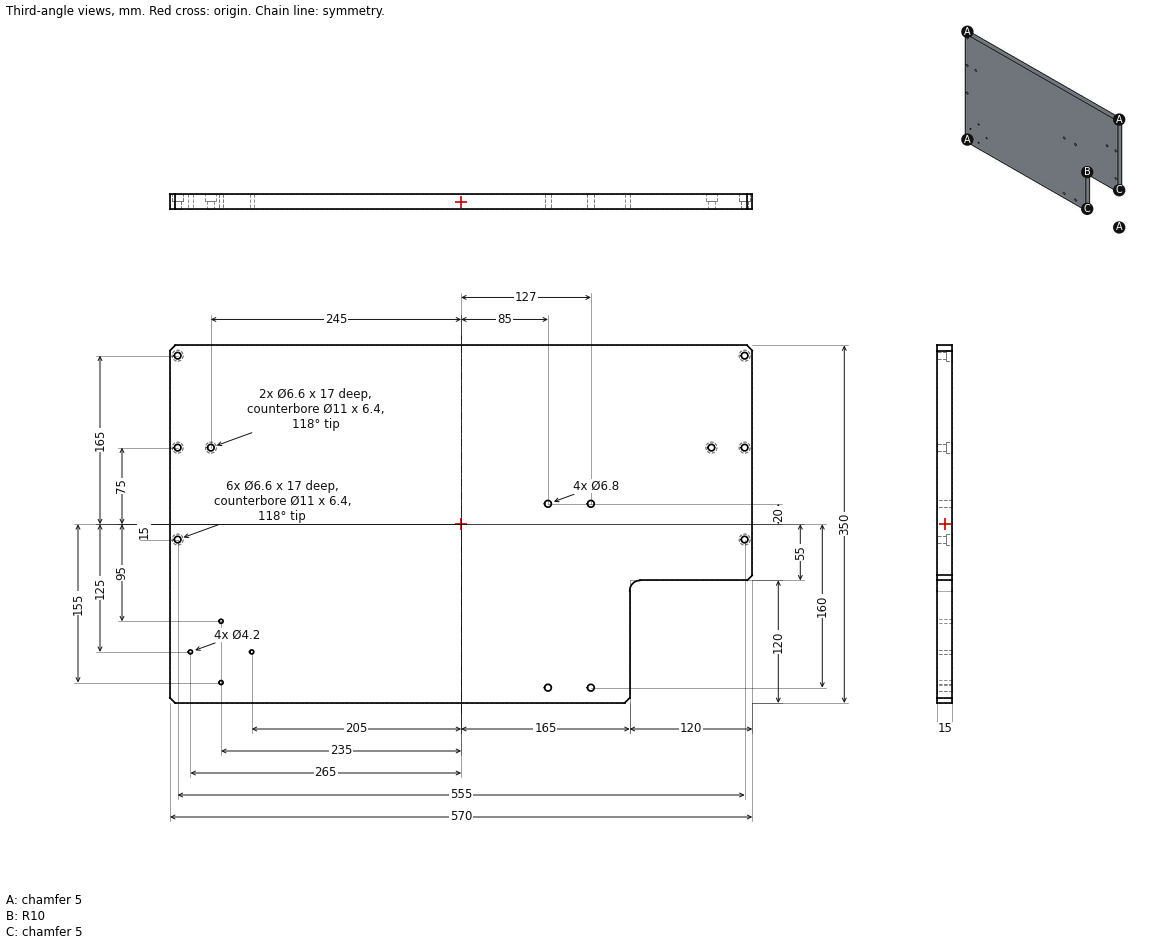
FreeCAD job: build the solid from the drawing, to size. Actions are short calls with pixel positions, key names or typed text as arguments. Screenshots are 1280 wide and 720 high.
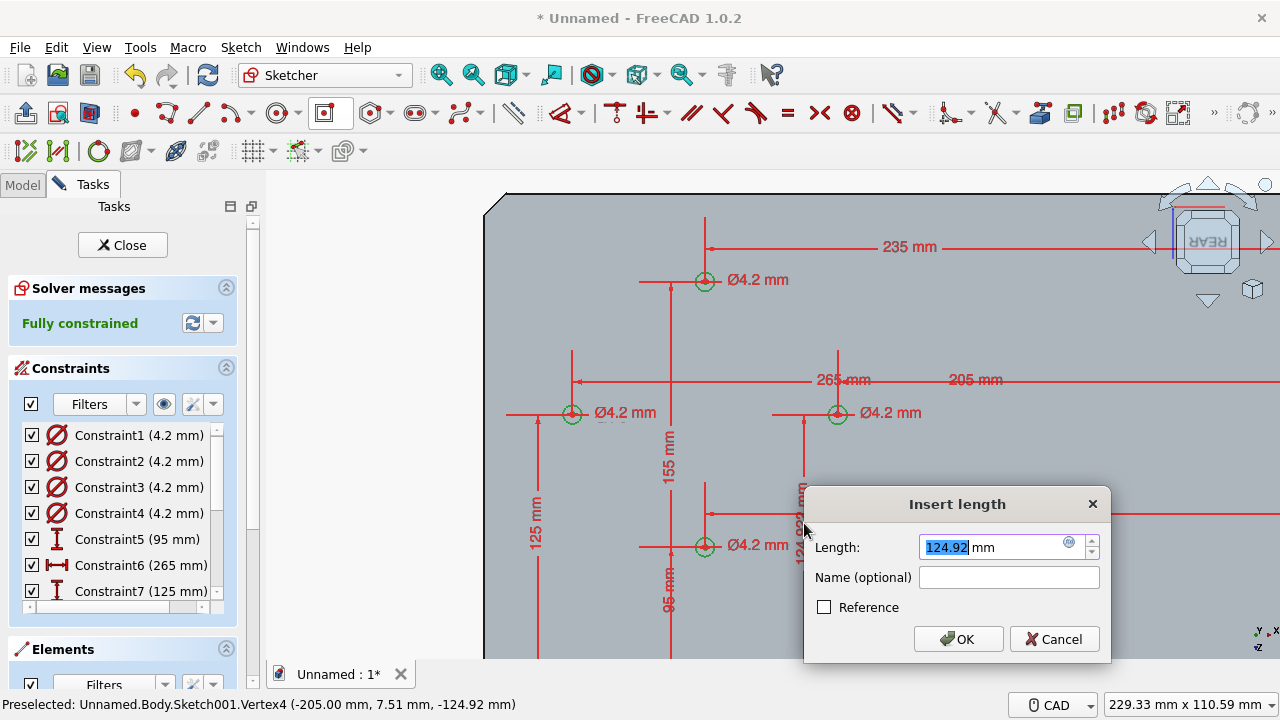
text(125)
key(Return)
key(Escape)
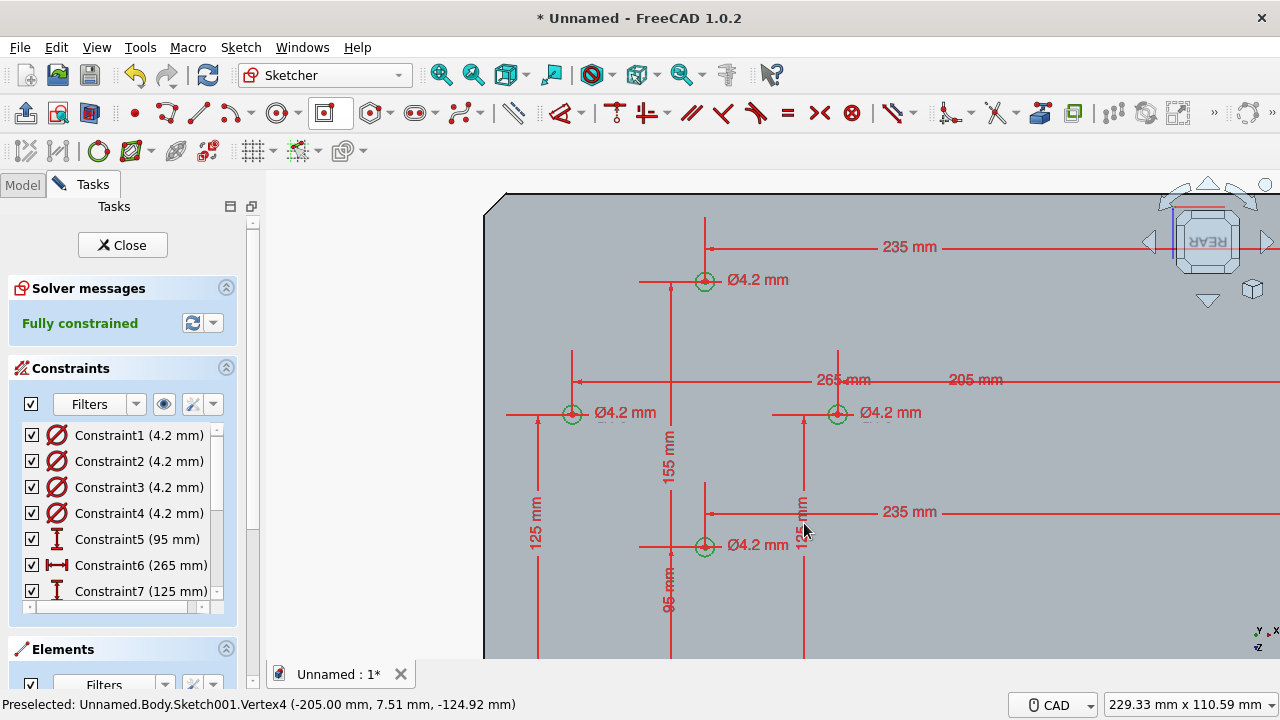
click(123, 245)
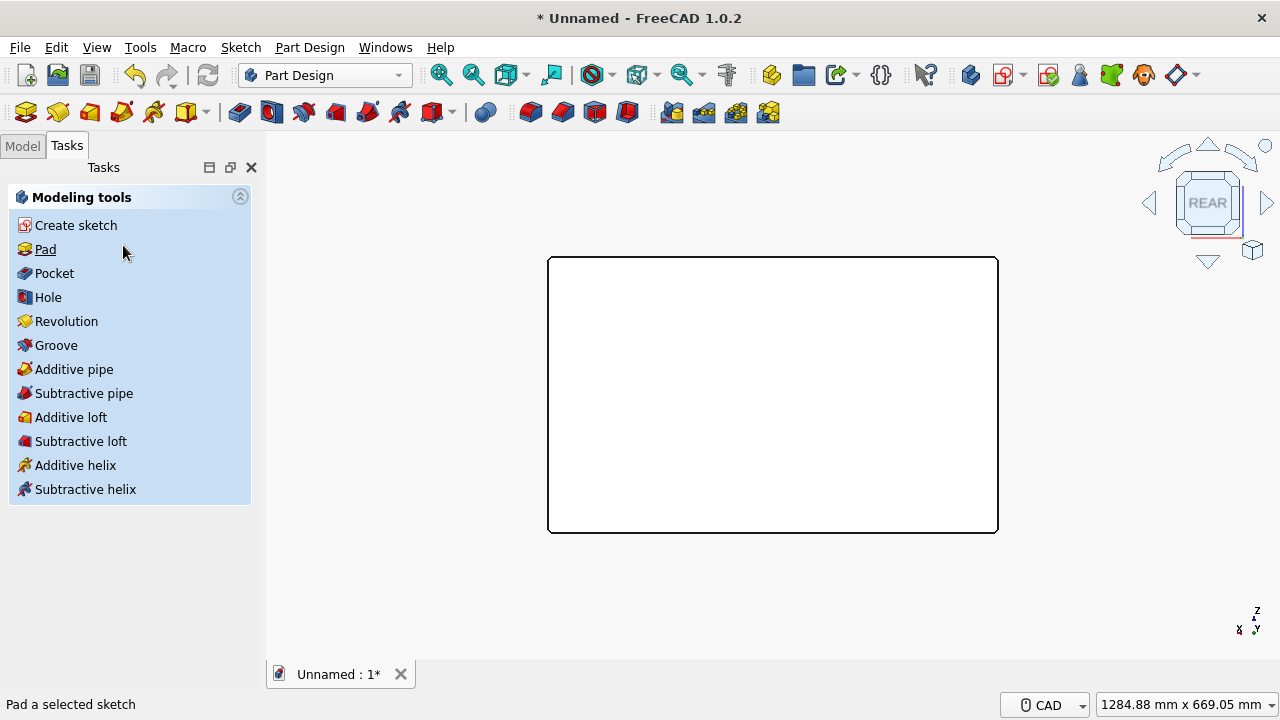
click(240, 112)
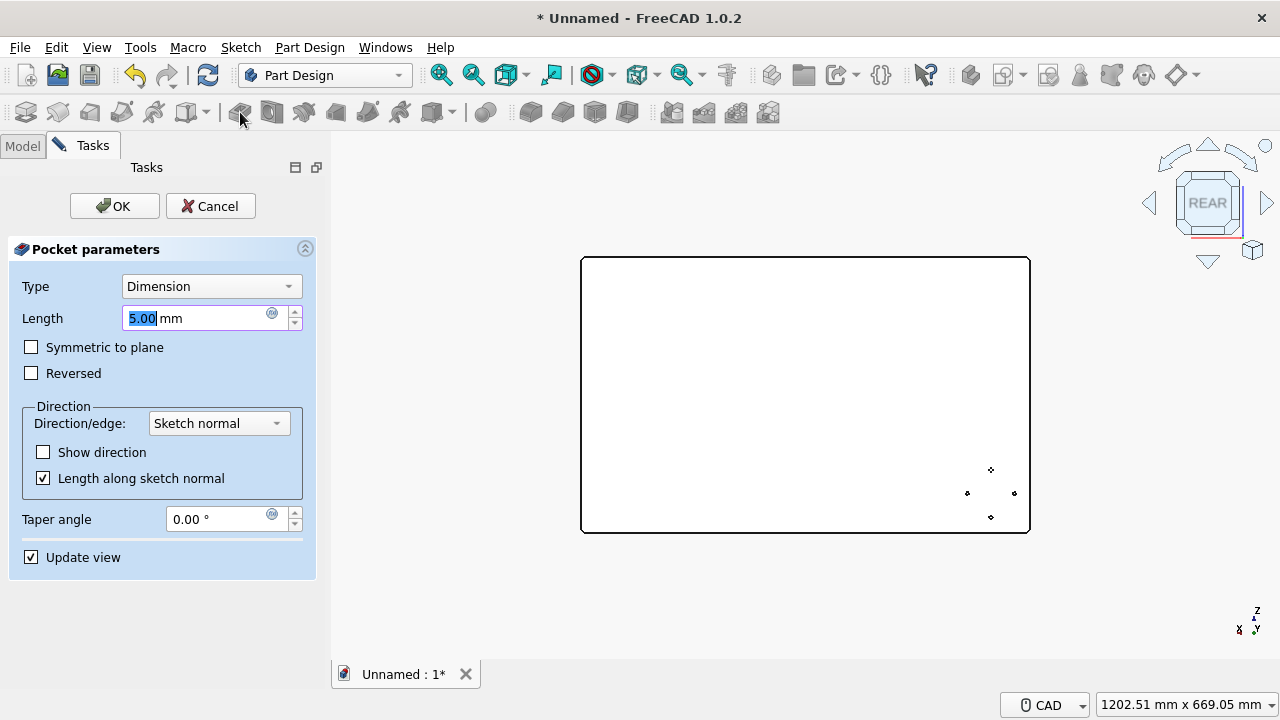
click(212, 286)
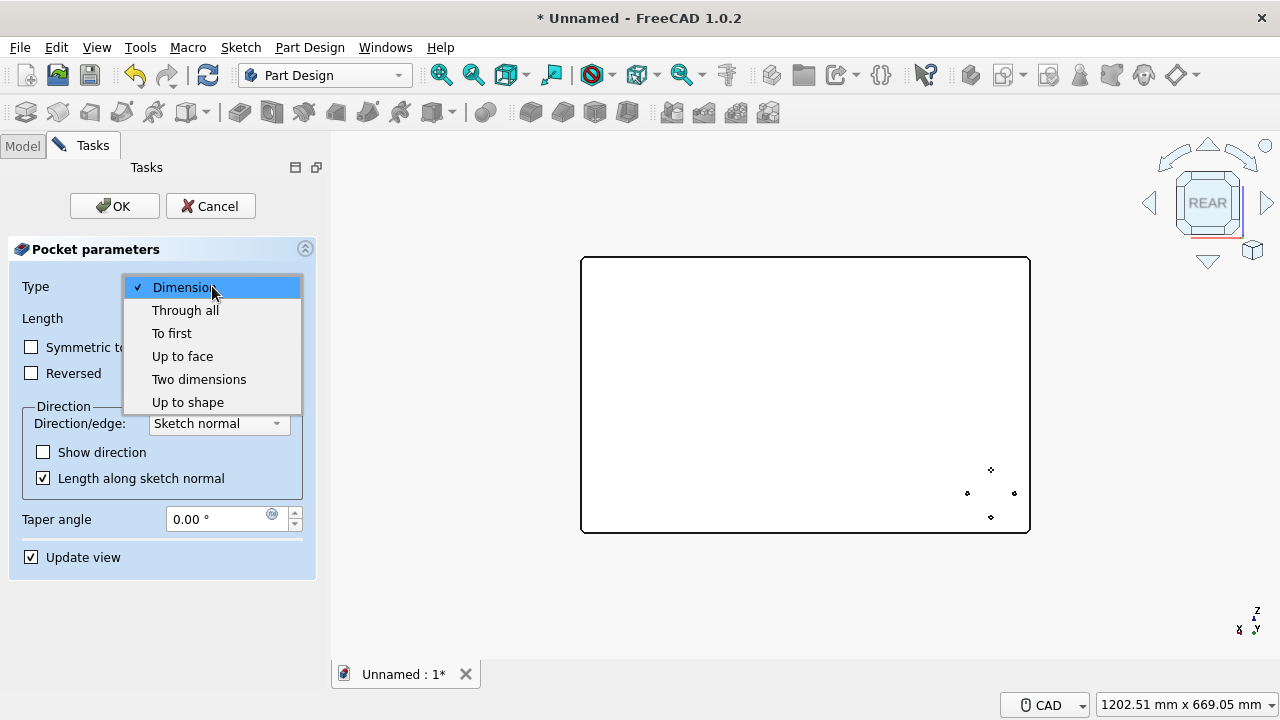
click(212, 310)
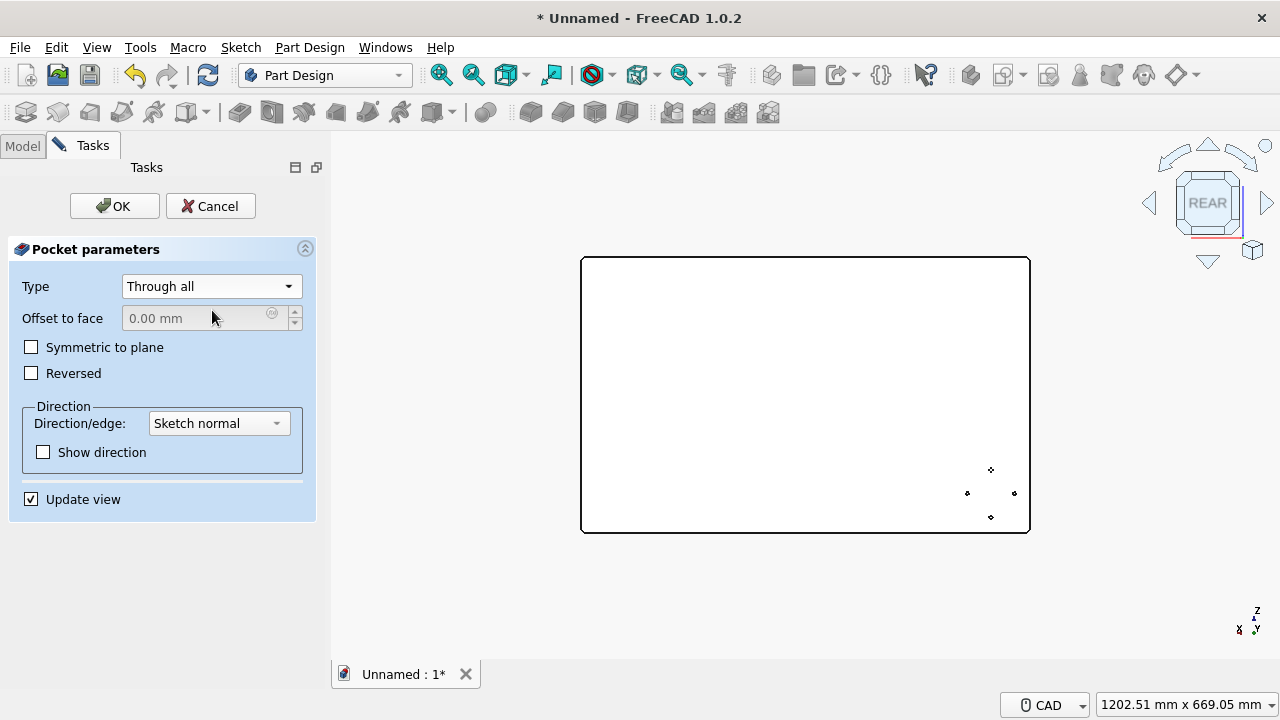
click(115, 206)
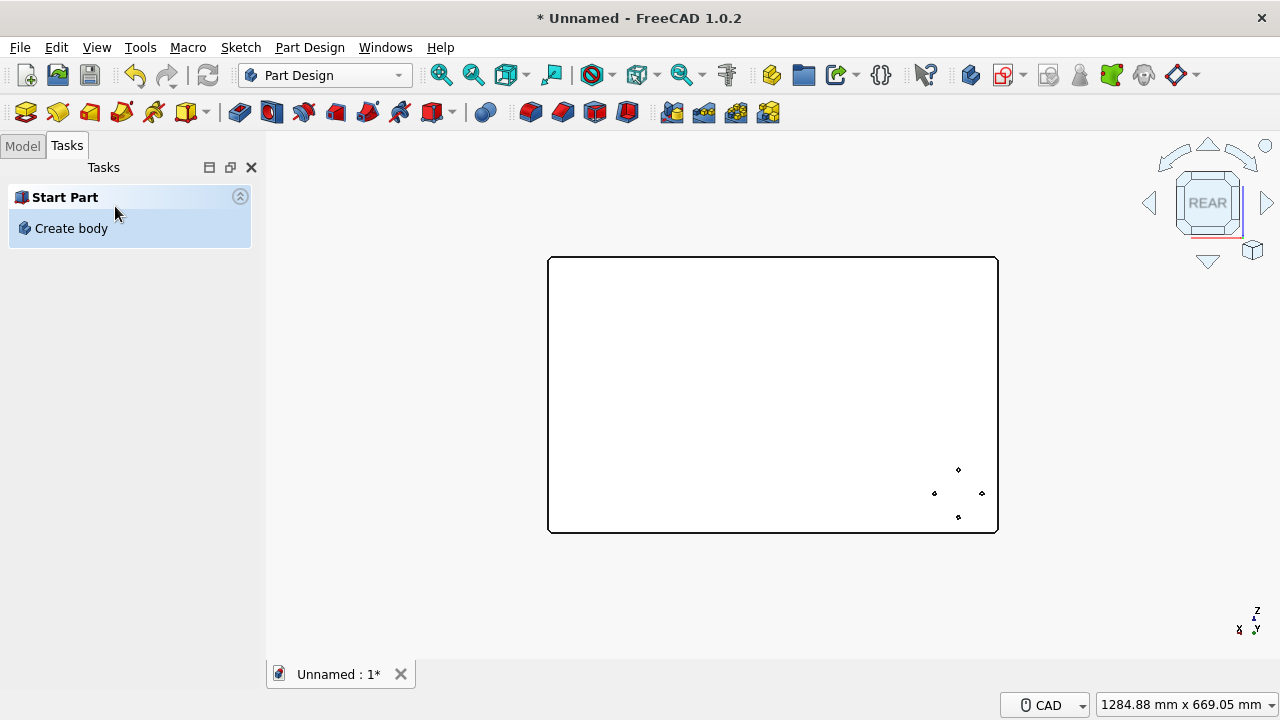
click(709, 394)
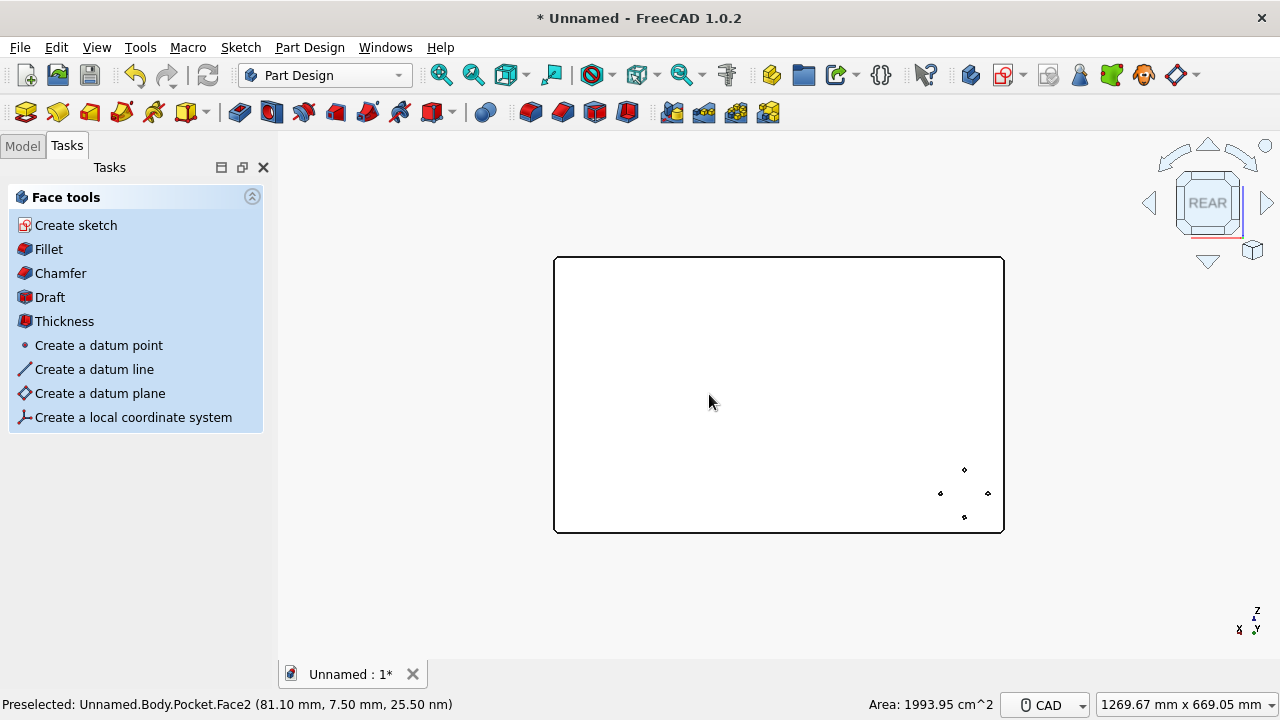
click(1004, 76)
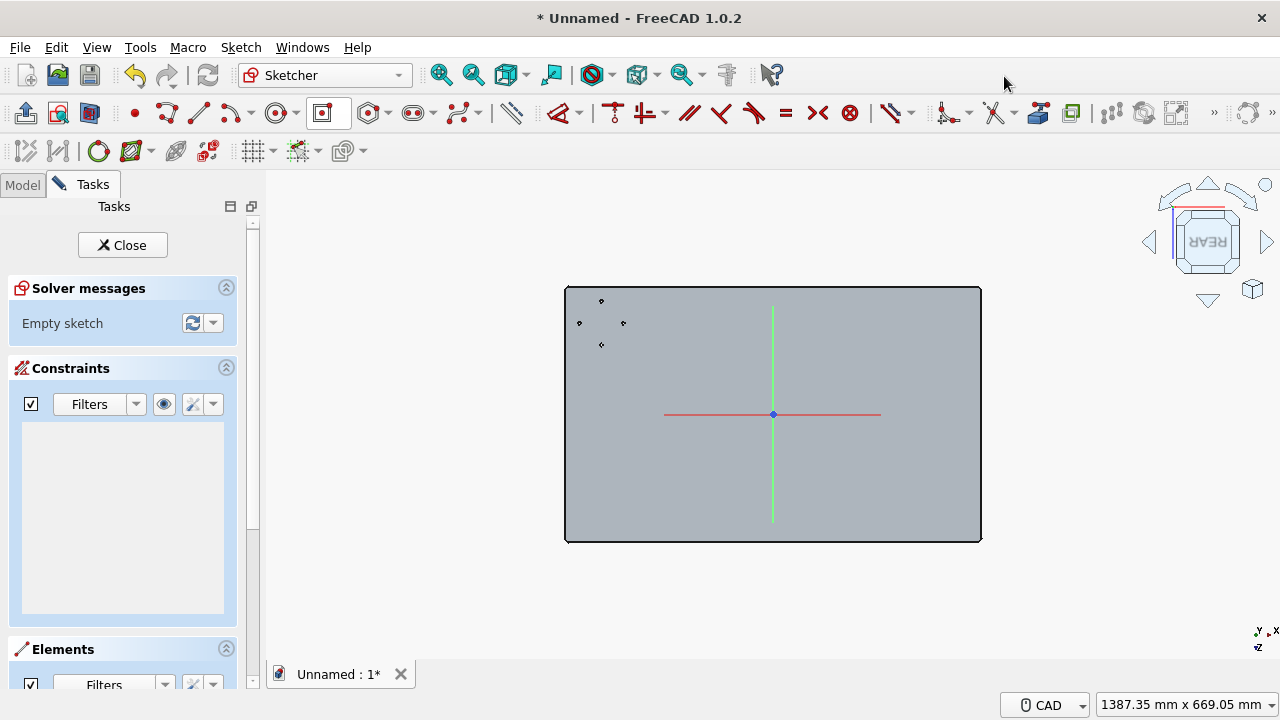
scroll(915, 322, up, 4)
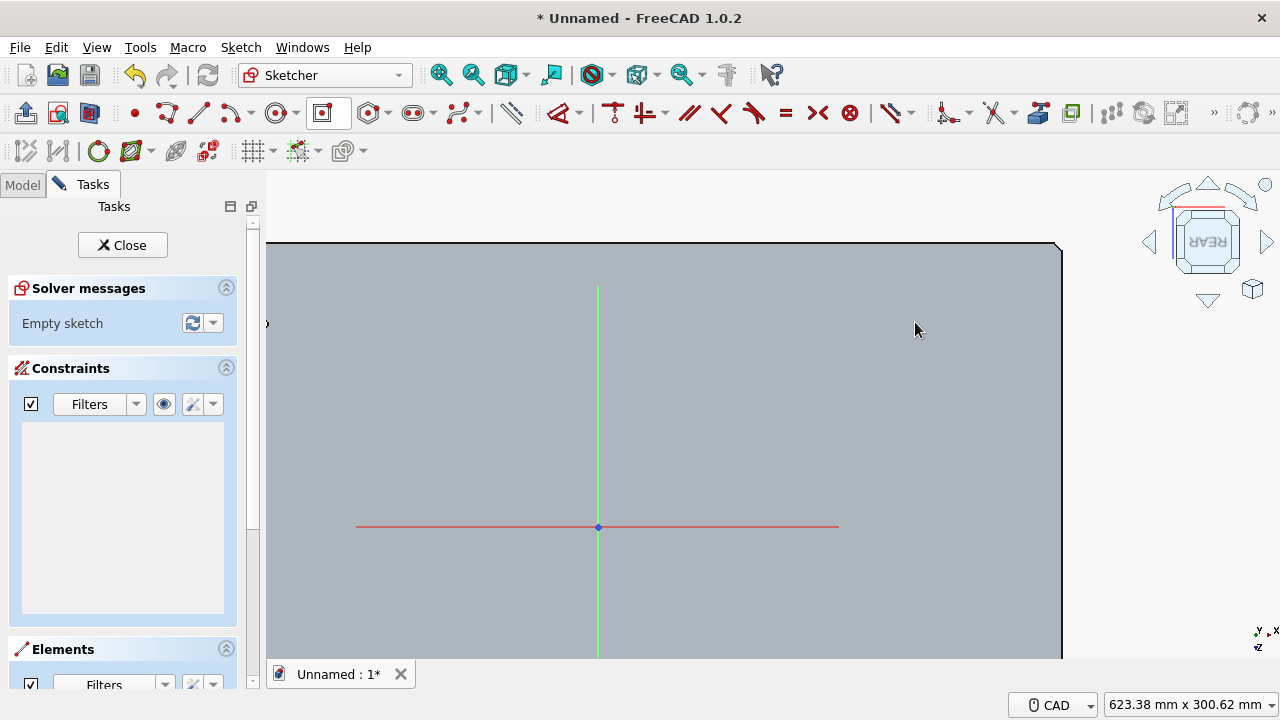
click(276, 114)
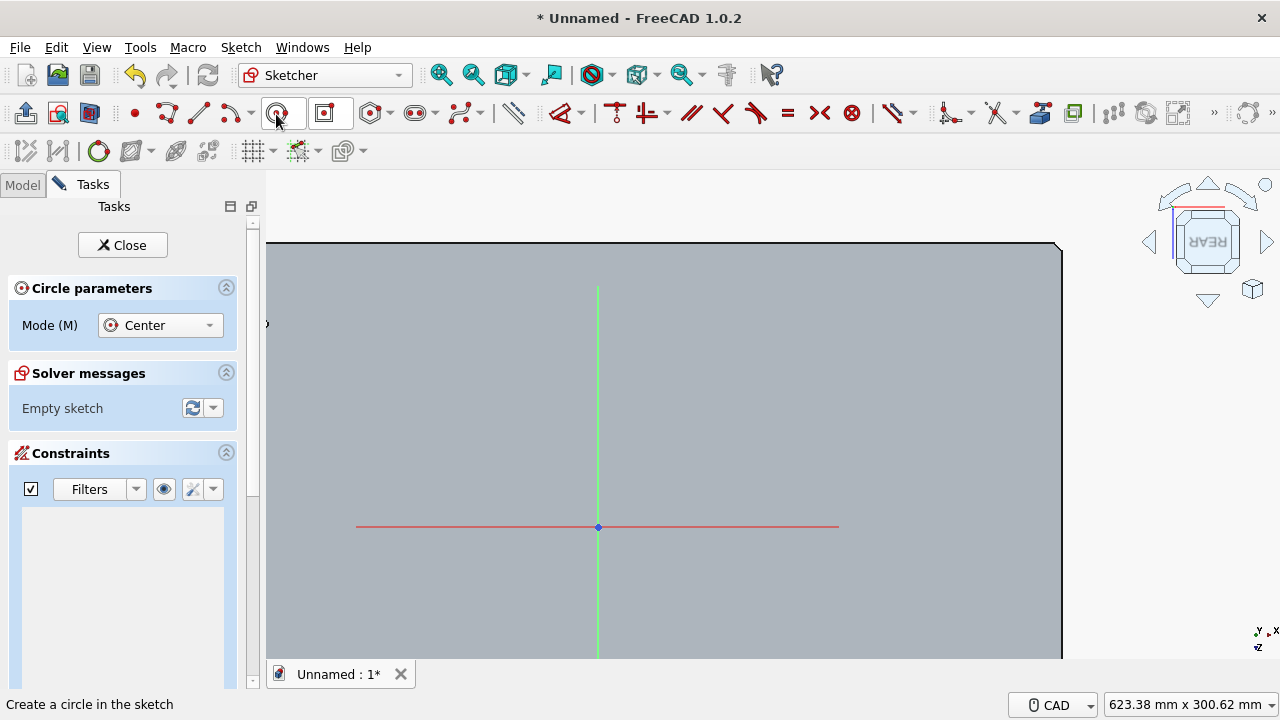
scroll(736, 560, up, 8)